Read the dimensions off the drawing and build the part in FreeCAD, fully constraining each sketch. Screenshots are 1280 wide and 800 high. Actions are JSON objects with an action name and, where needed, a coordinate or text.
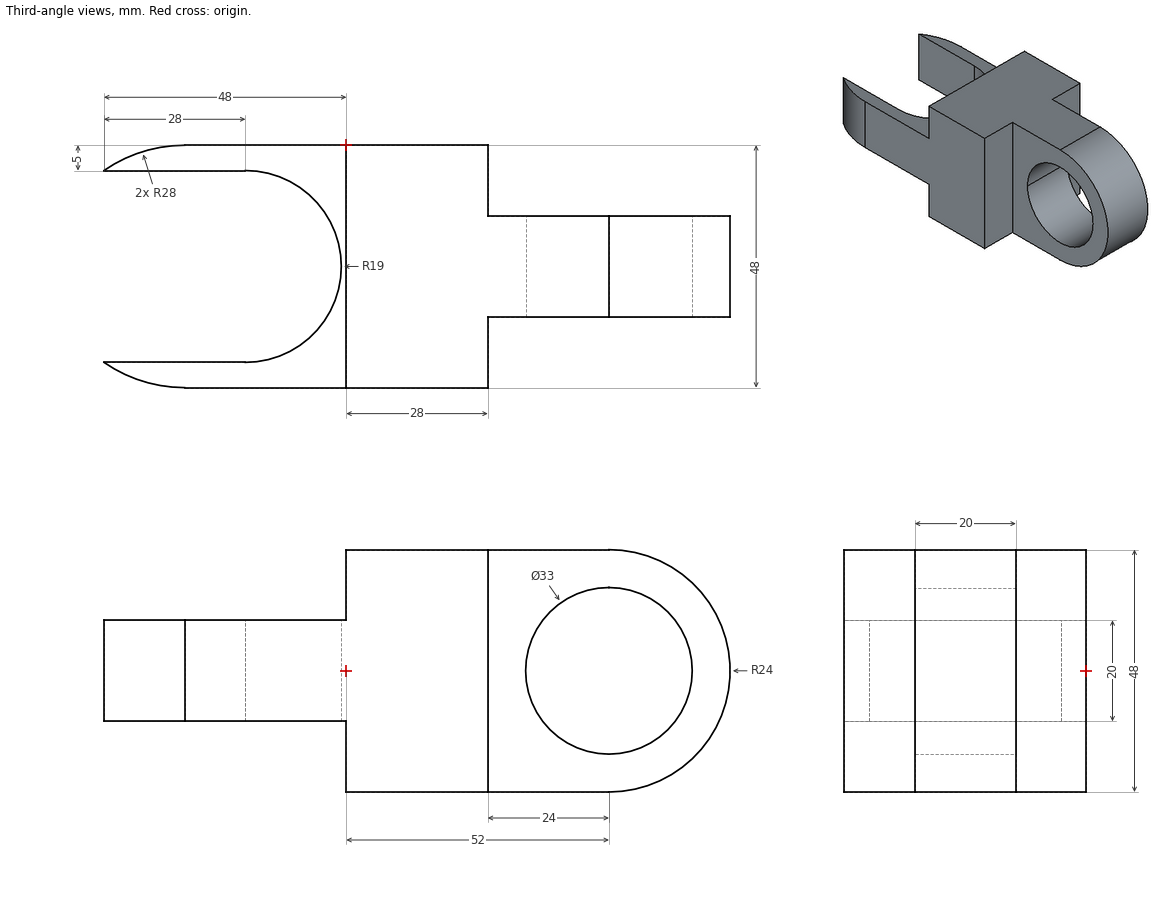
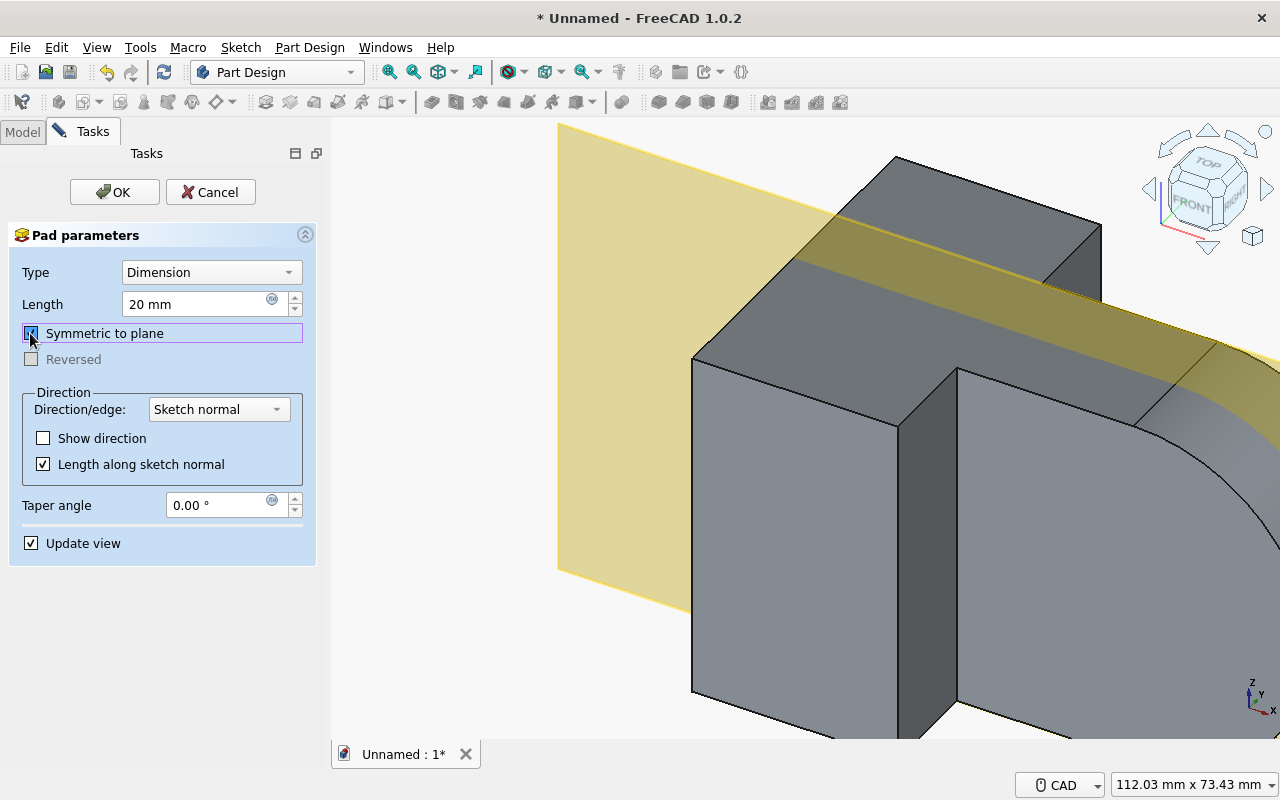
{"action": "left_click", "coordinate": [115, 192]}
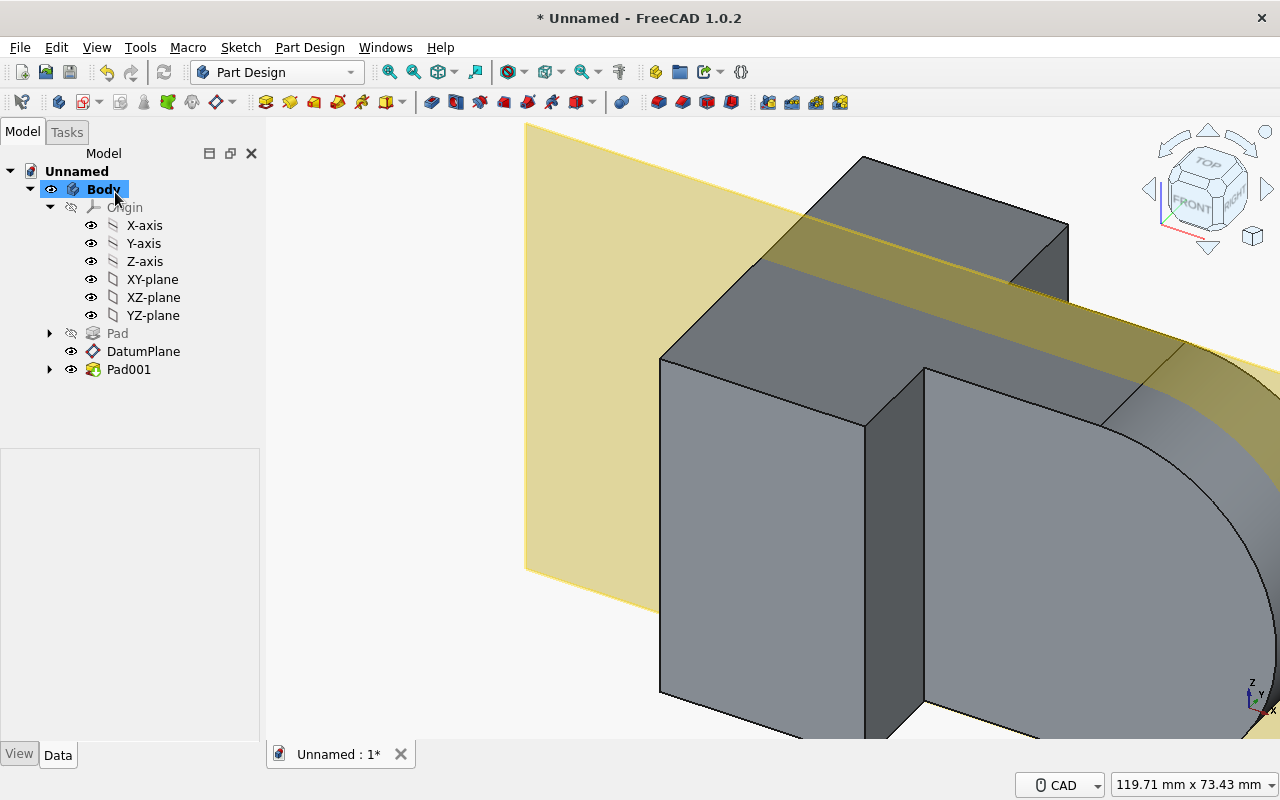
{"action": "left_click", "coordinate": [116, 351]}
{"action": "key", "text": "space"}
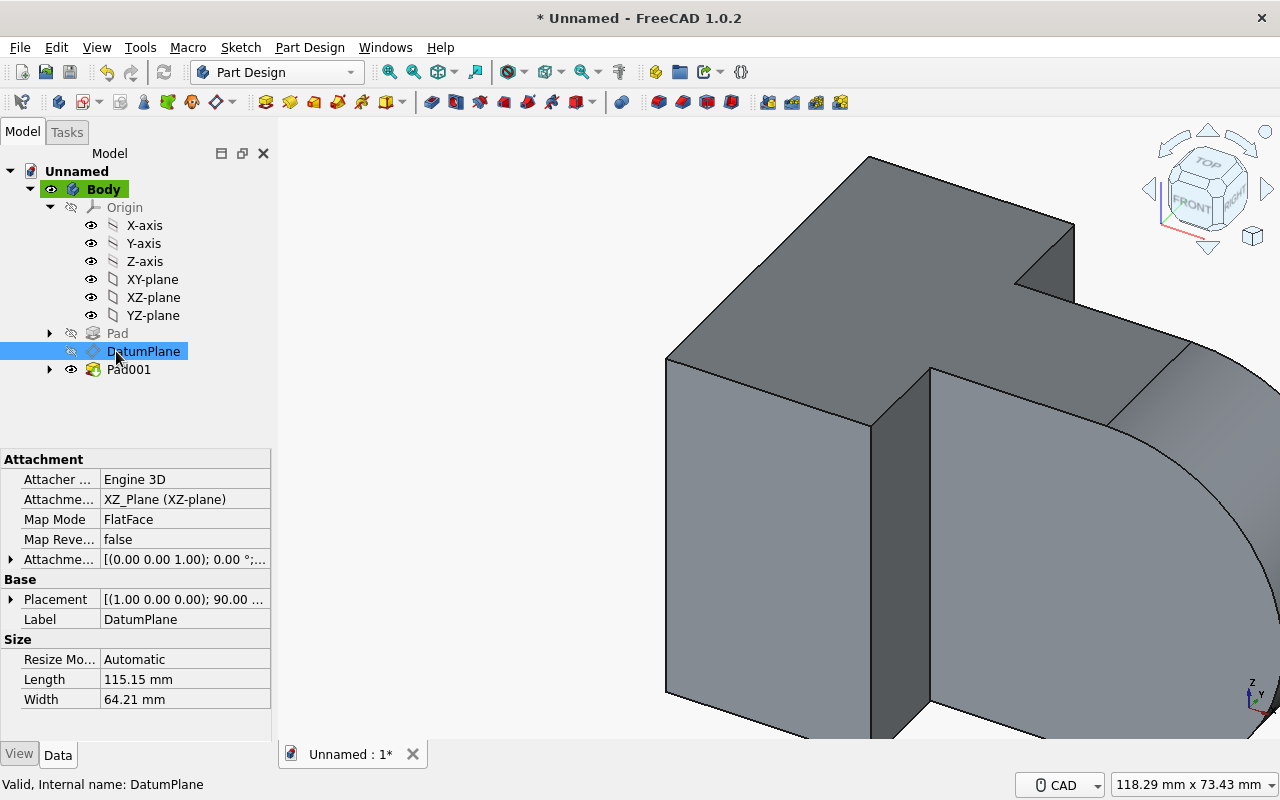
{"action": "left_click", "coordinate": [390, 72]}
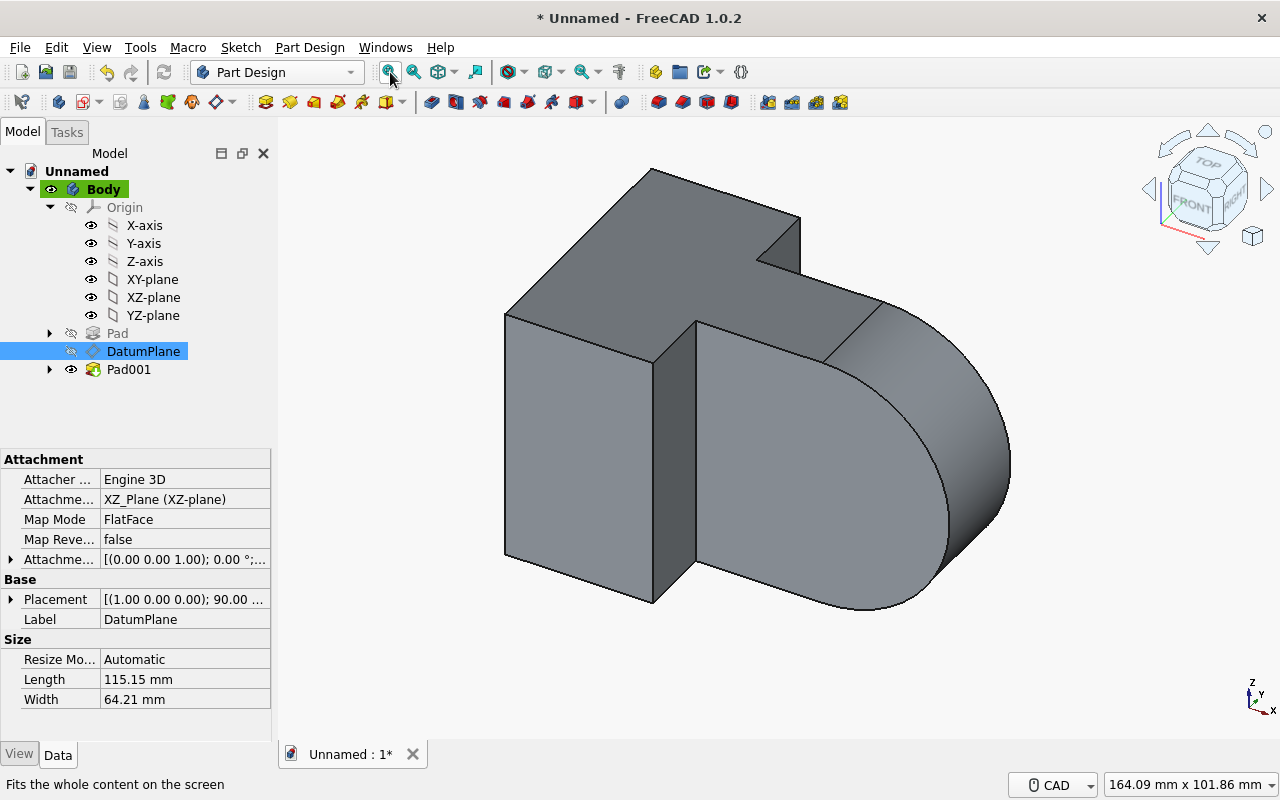
{"action": "key", "text": "4"}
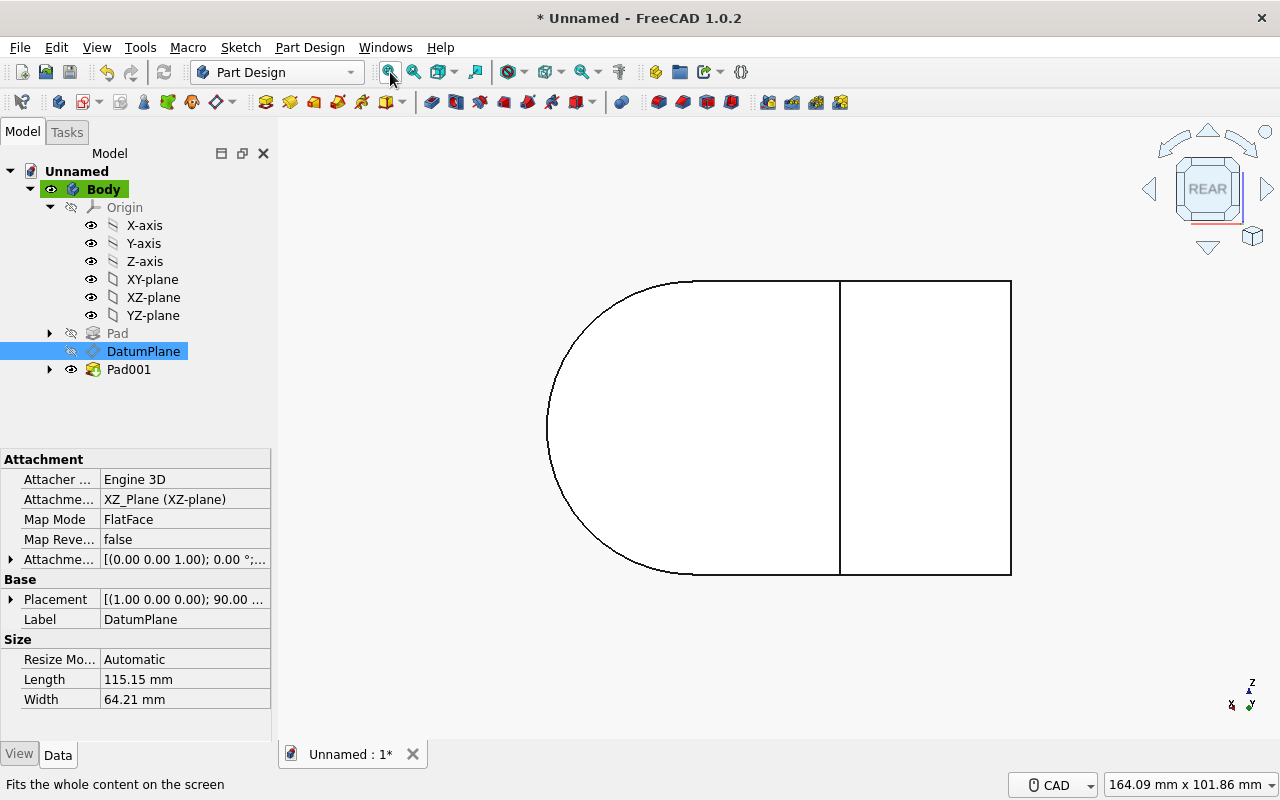
{"action": "left_click", "coordinate": [693, 427]}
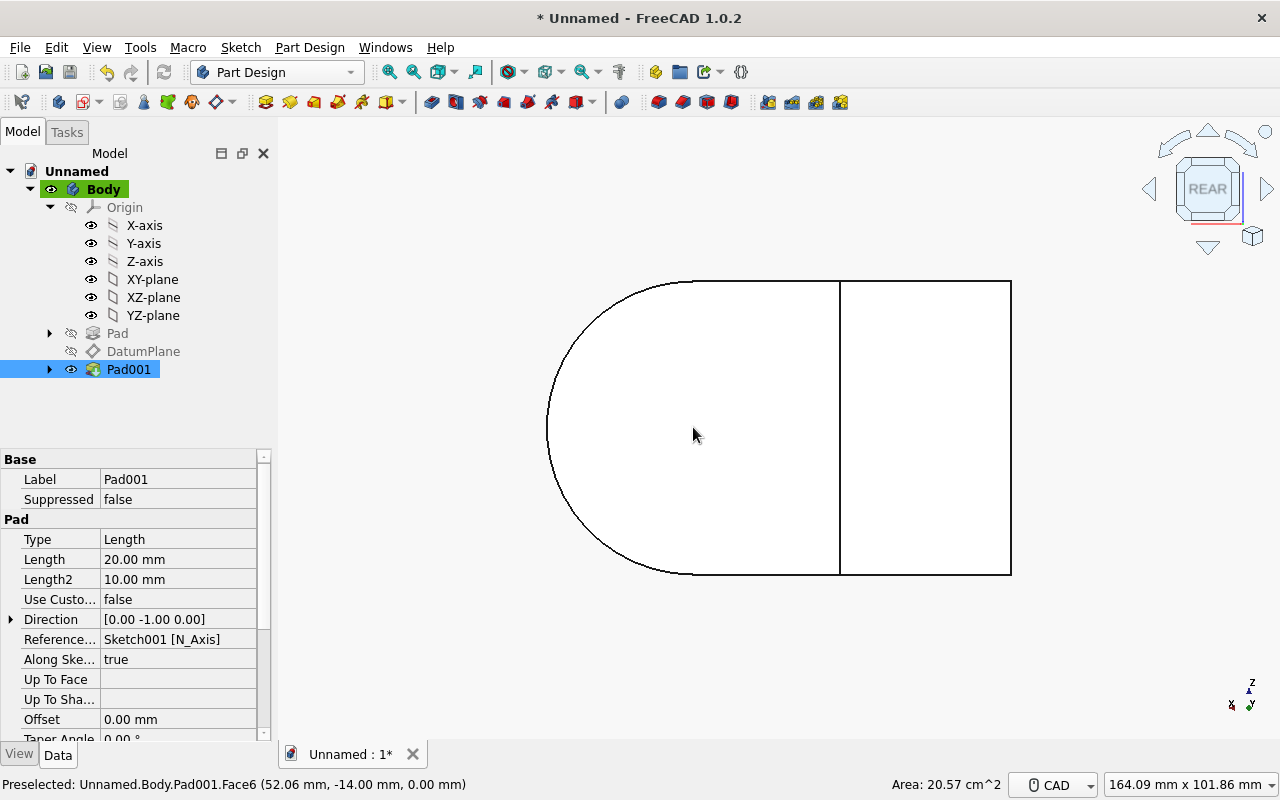
{"action": "left_click", "coordinate": [84, 102]}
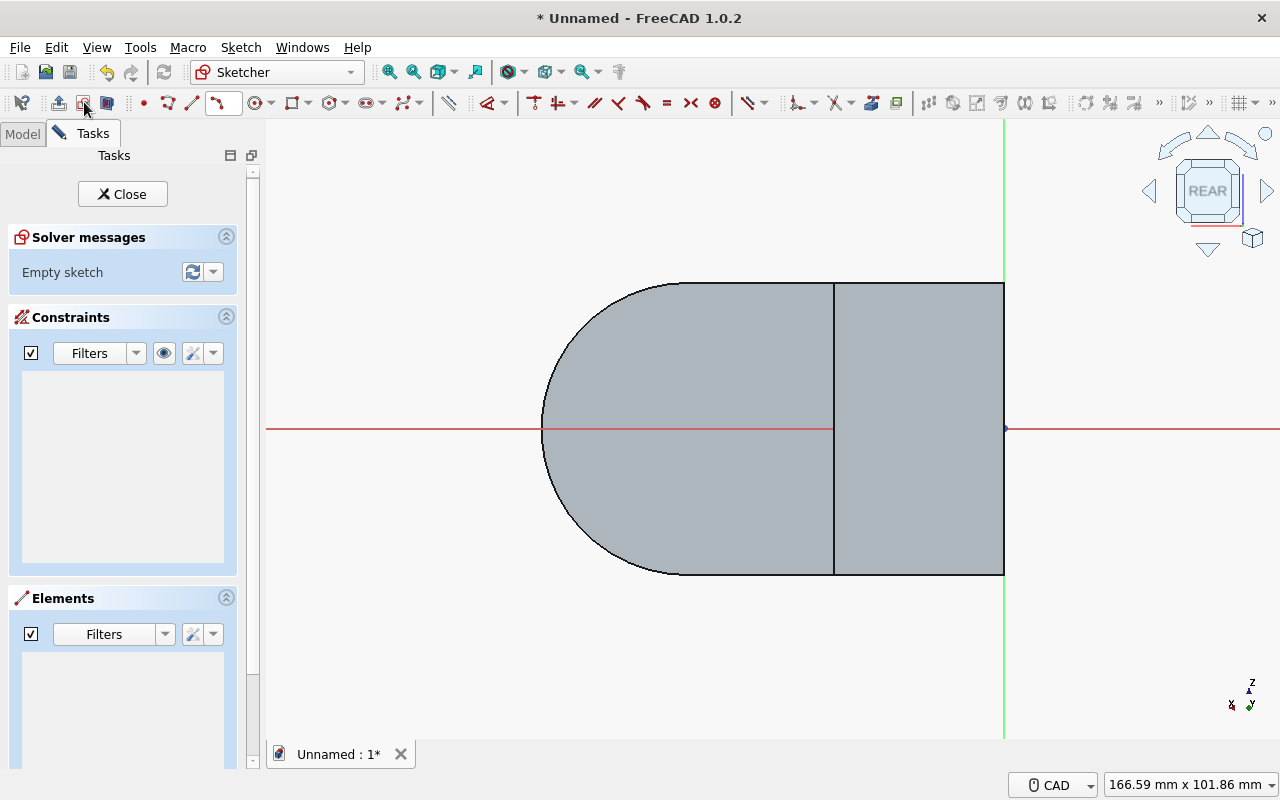
{"action": "scroll", "coordinate": [981, 429], "scroll_direction": "up", "scroll_amount": 2}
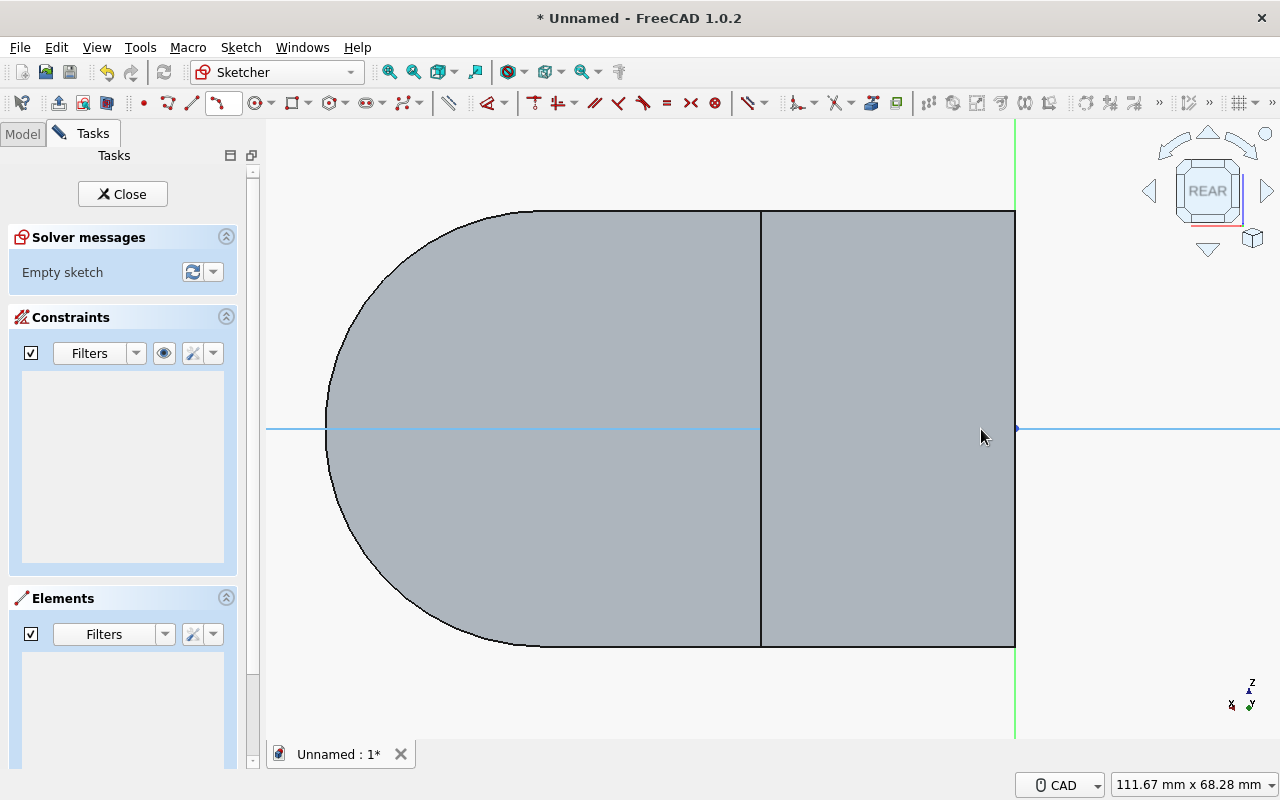
{"action": "left_click", "coordinate": [256, 104]}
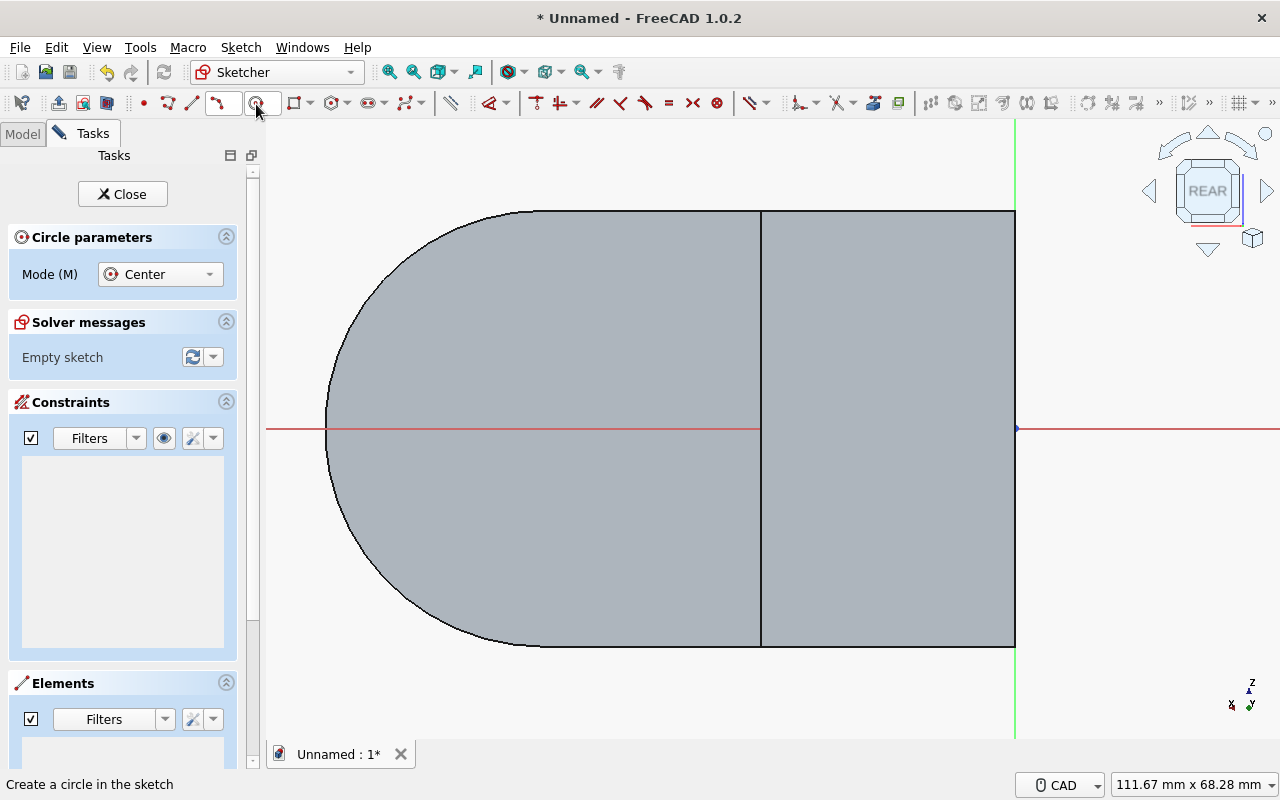
{"action": "left_click", "coordinate": [543, 429]}
{"action": "mouse_move", "coordinate": [649, 323]}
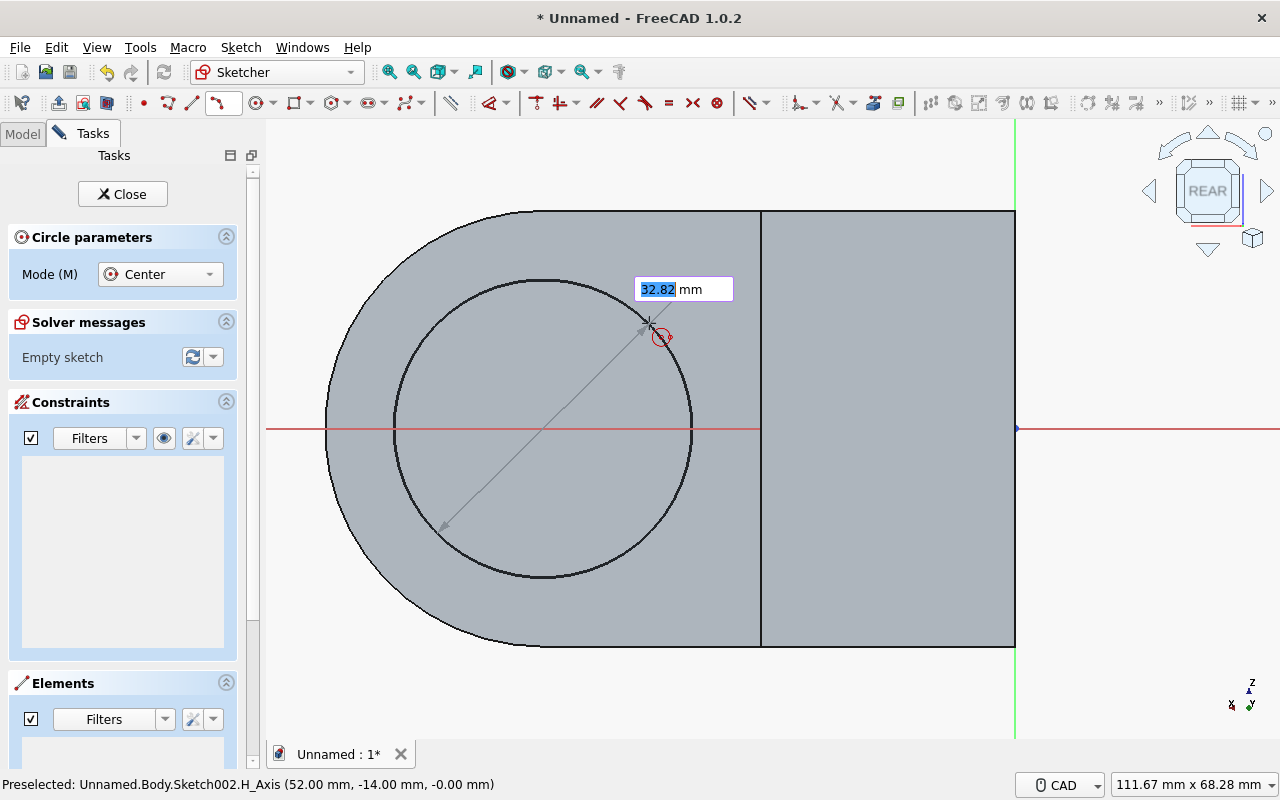
{"action": "type", "text": "33"}
{"action": "key", "text": "Return"}
{"action": "key", "text": "Escape"}